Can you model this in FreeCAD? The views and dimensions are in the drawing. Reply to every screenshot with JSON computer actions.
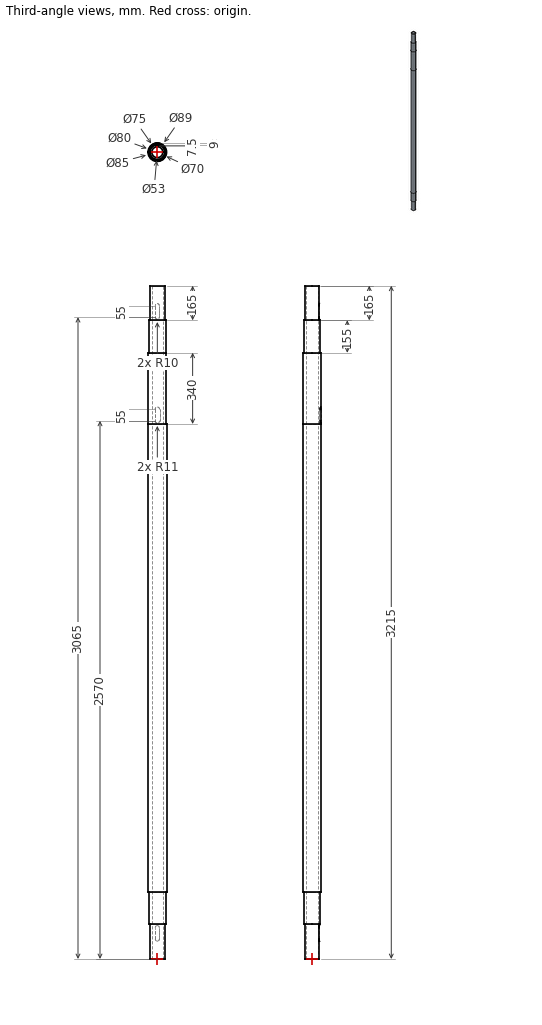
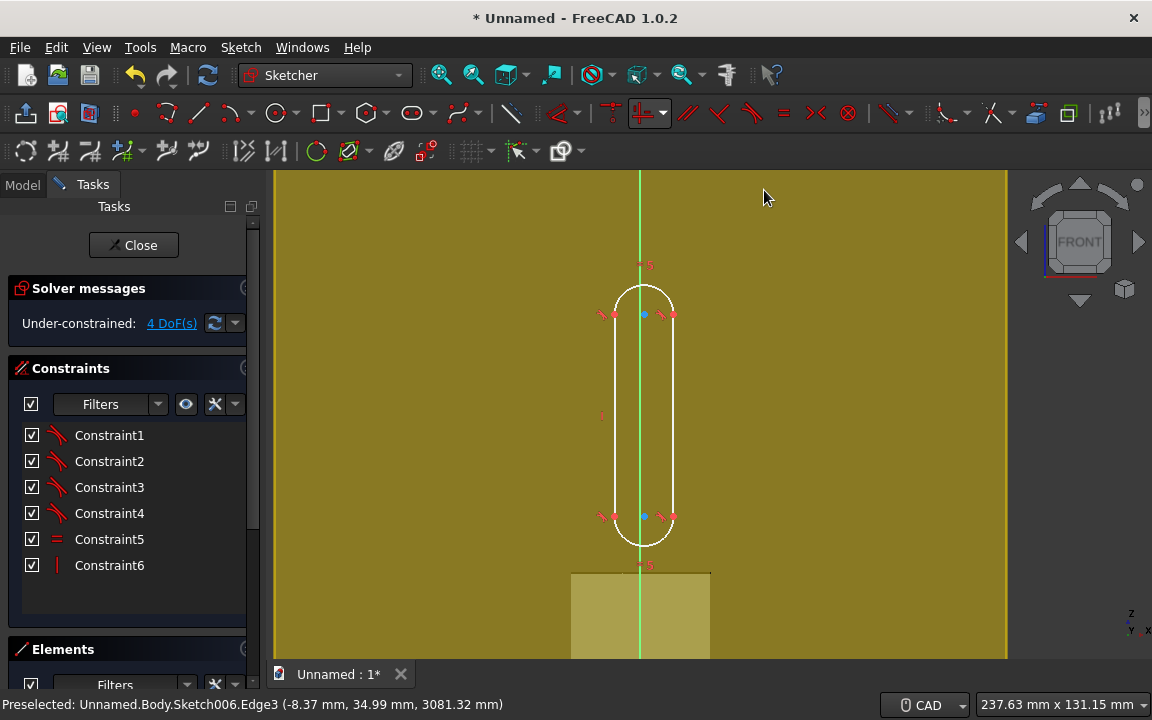
{"action": "left_click", "coordinate": [644, 517]}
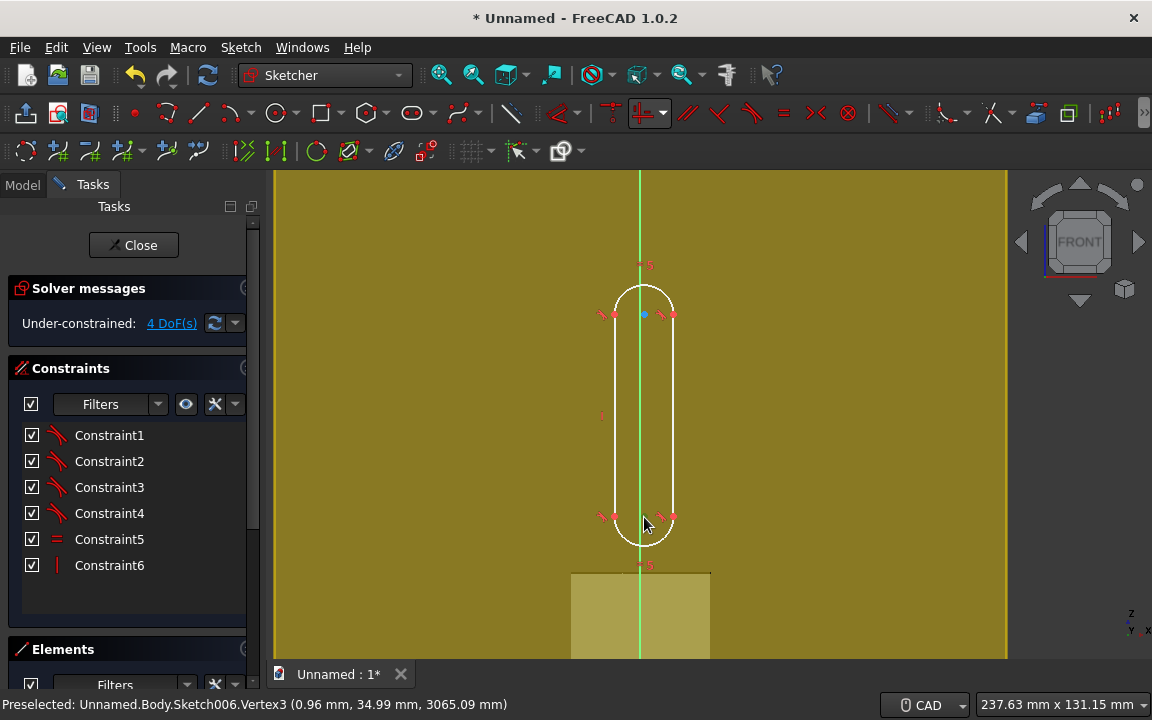
{"action": "left_click", "coordinate": [640, 600]}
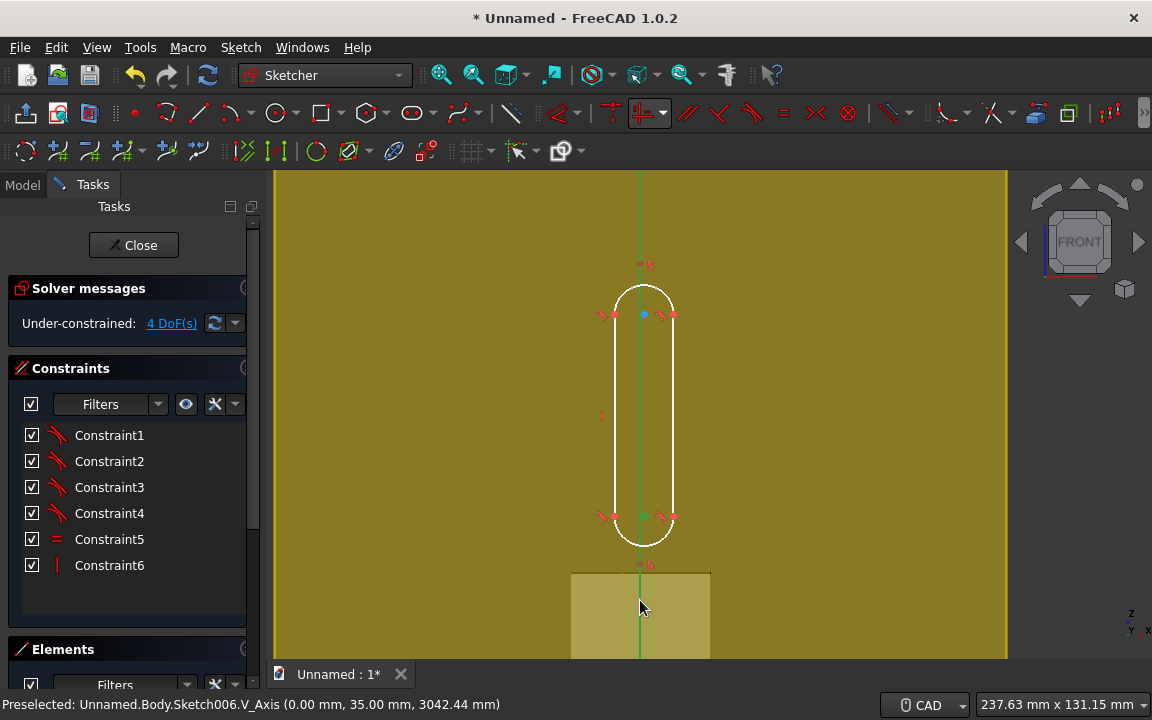
{"action": "left_click", "coordinate": [612, 114]}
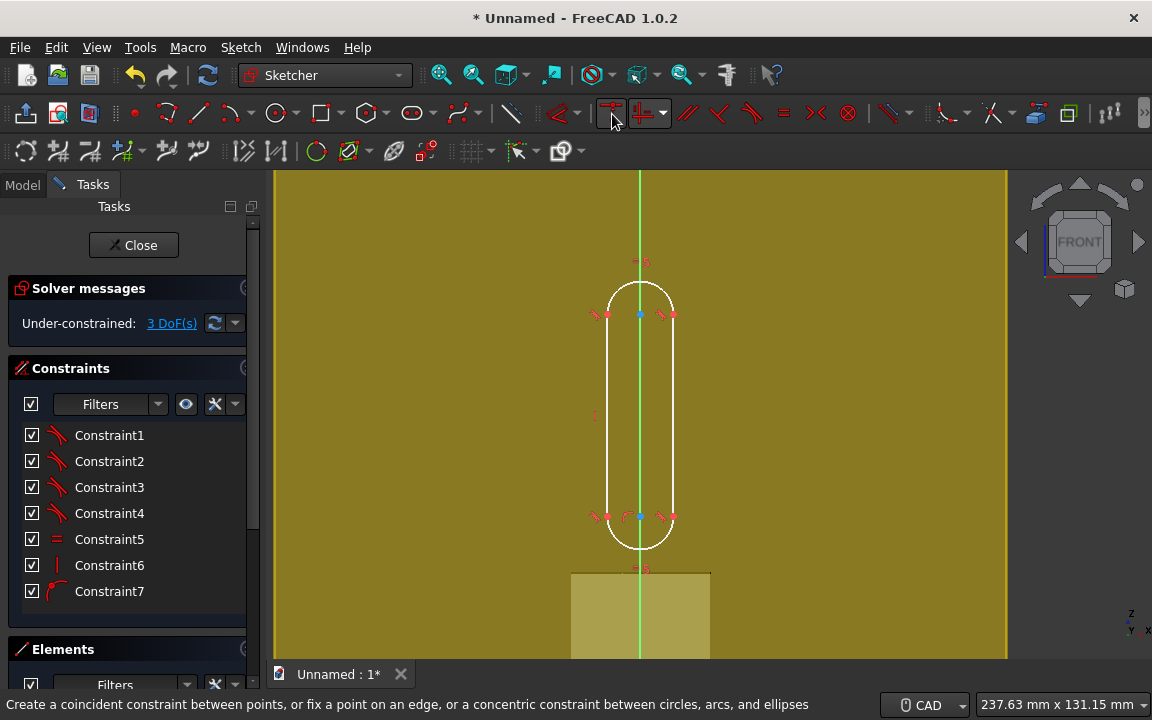
{"action": "left_click", "coordinate": [558, 114]}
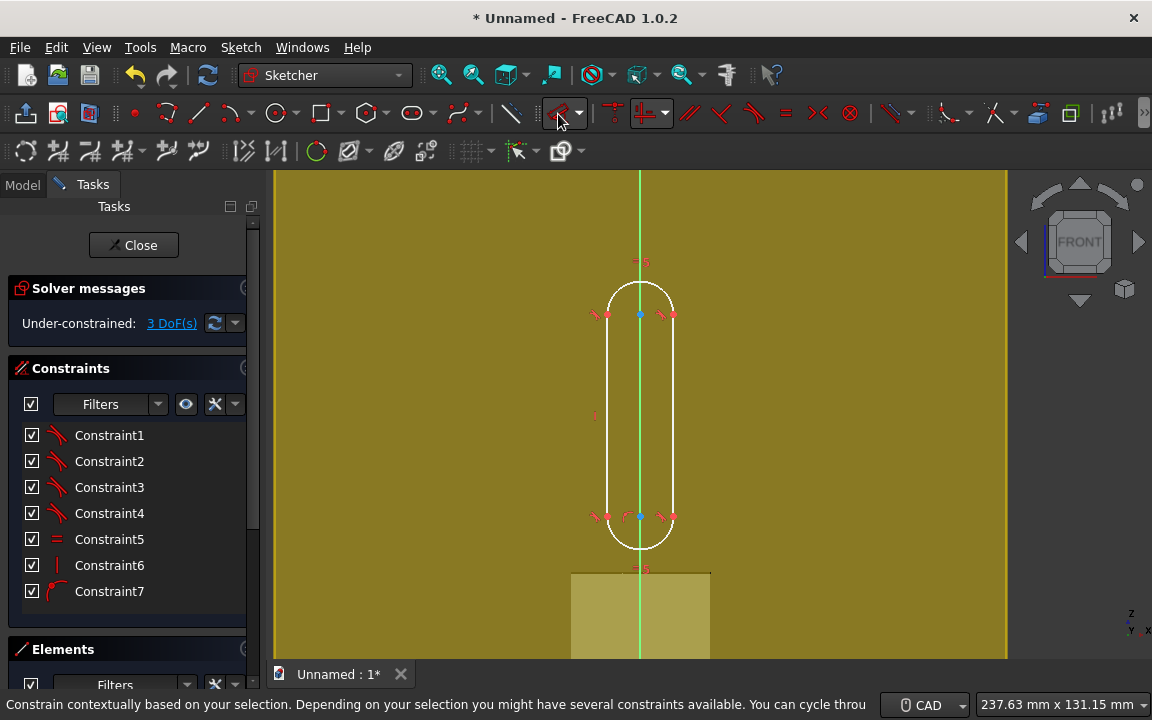
{"action": "left_click", "coordinate": [621, 543]}
{"action": "left_click", "coordinate": [602, 569]}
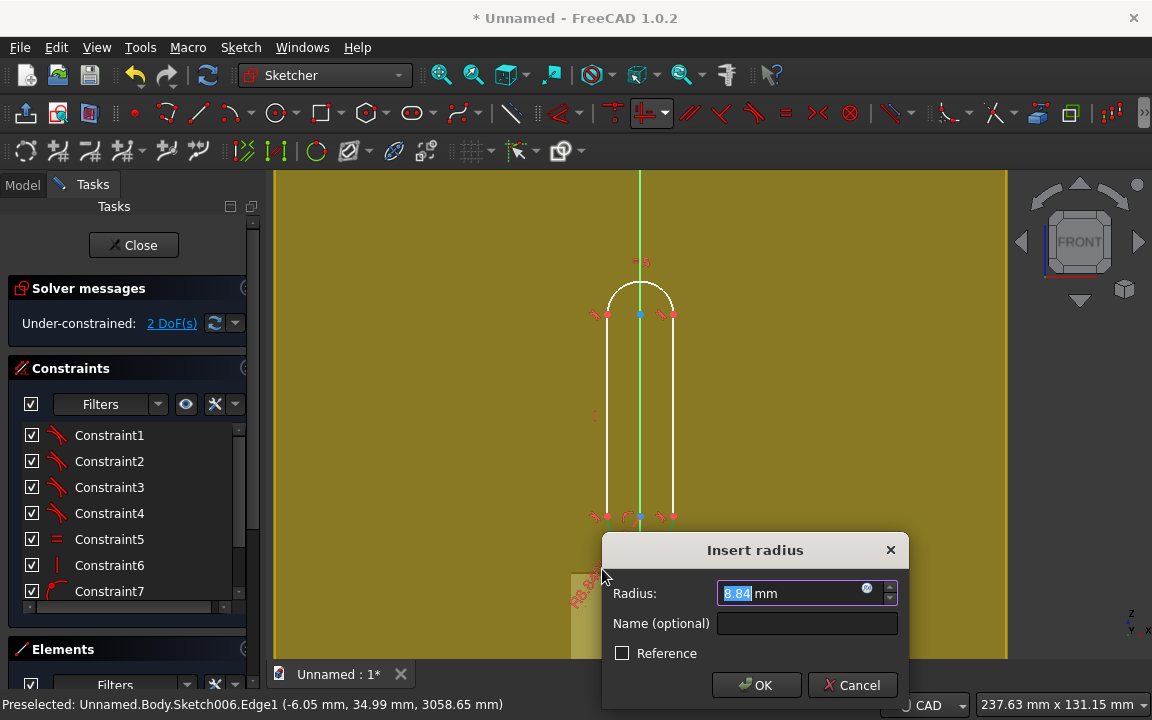
{"action": "type", "text": "10"}
{"action": "key", "text": "Return"}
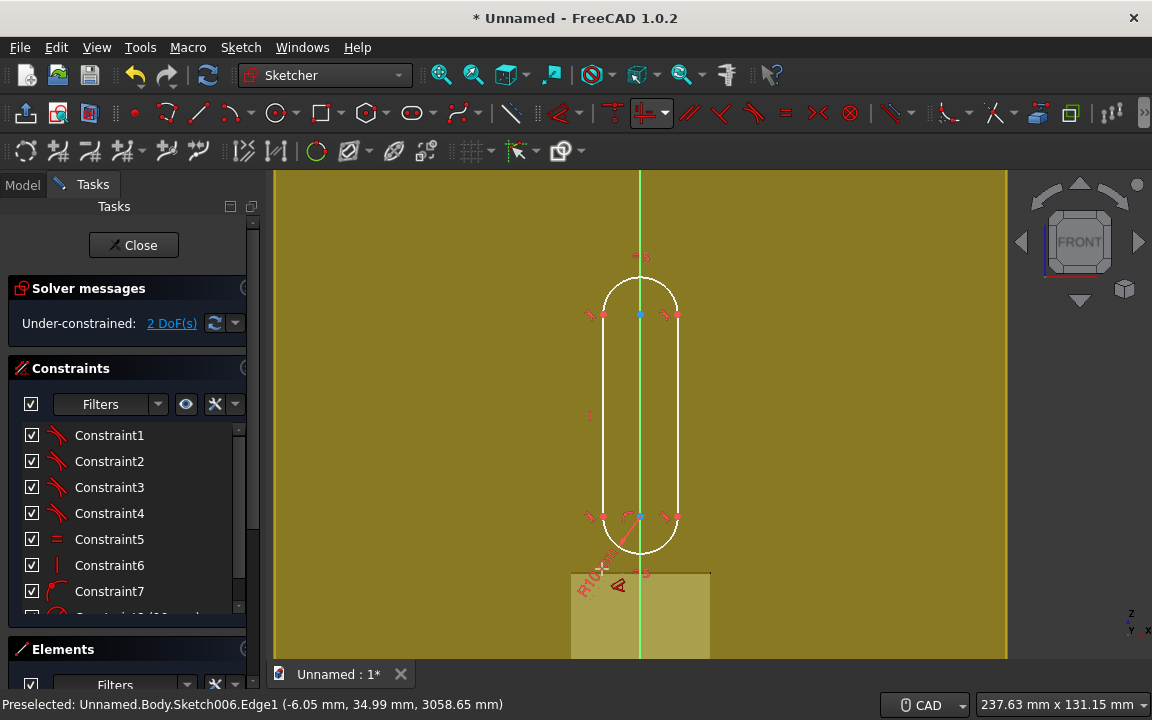
{"action": "left_click", "coordinate": [603, 456]}
{"action": "left_click", "coordinate": [569, 416]}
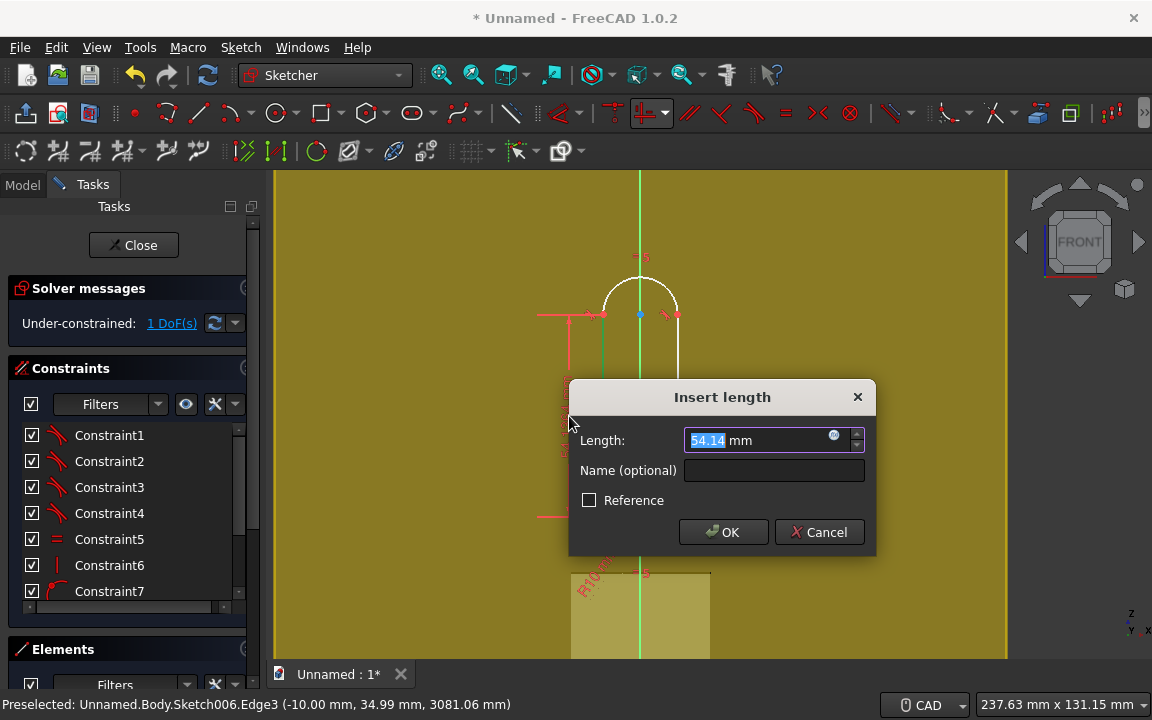
{"action": "type", "text": "55"}
{"action": "key", "text": "Return"}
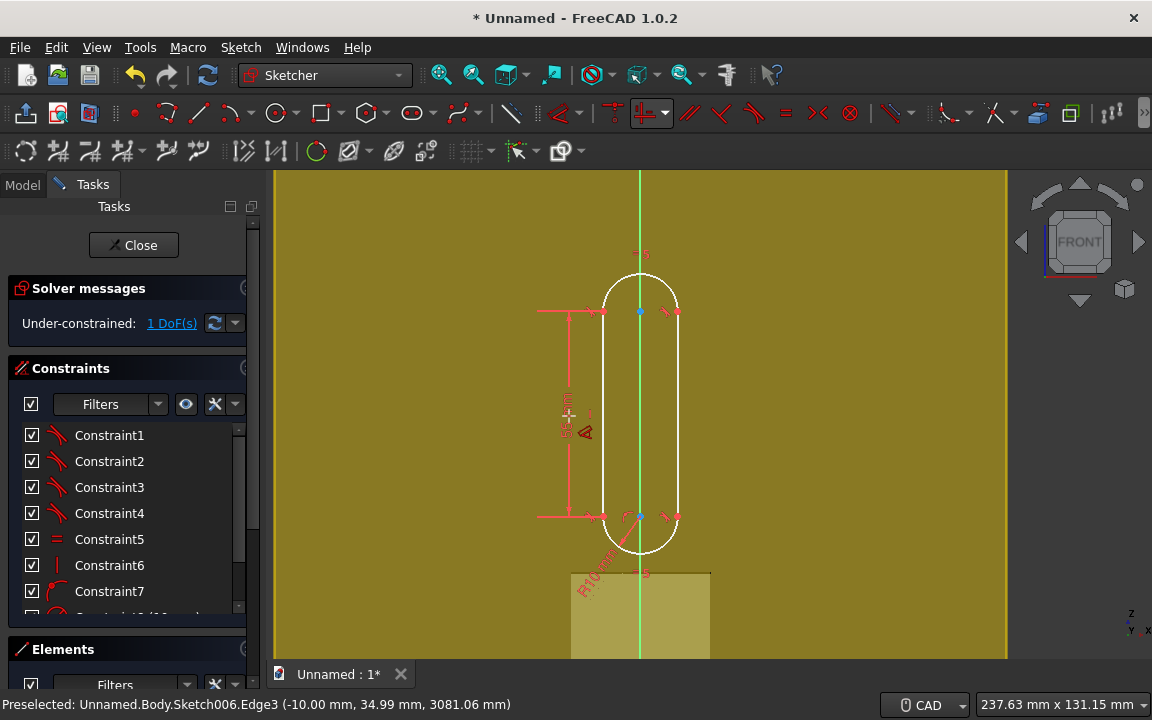
{"action": "left_click", "coordinate": [603, 517]}
{"action": "left_click", "coordinate": [569, 547]}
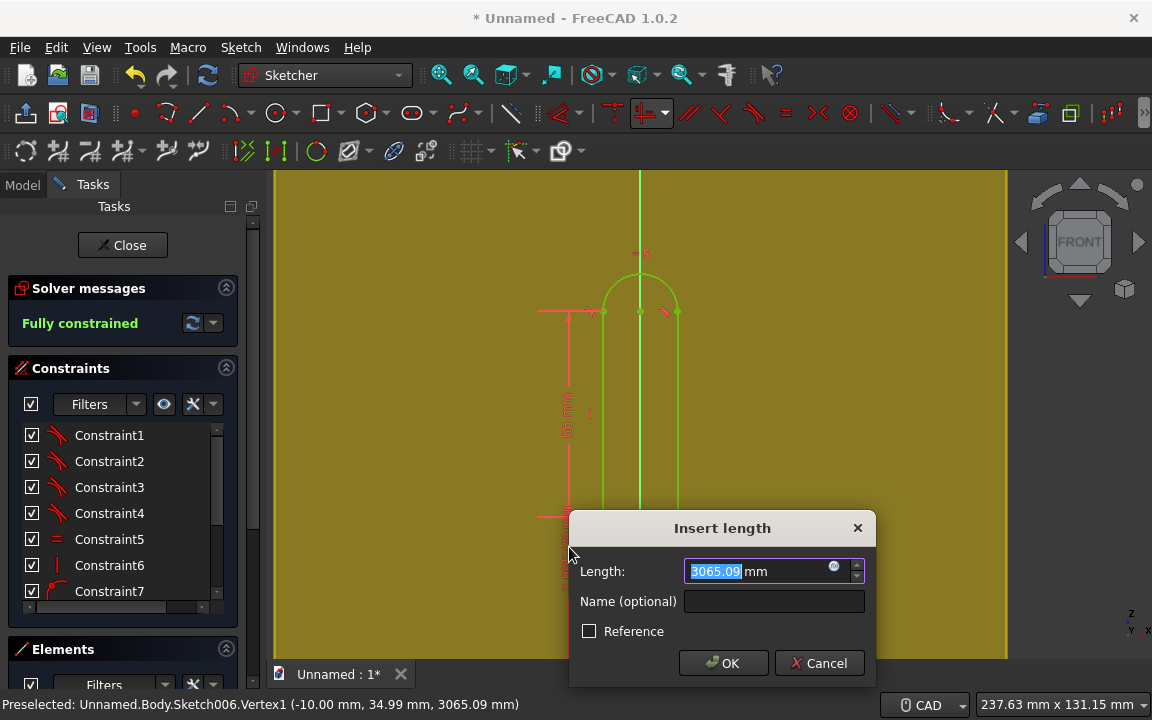
{"action": "type", "text": "3065"}
{"action": "key", "text": "Return"}
{"action": "key", "text": "Escape"}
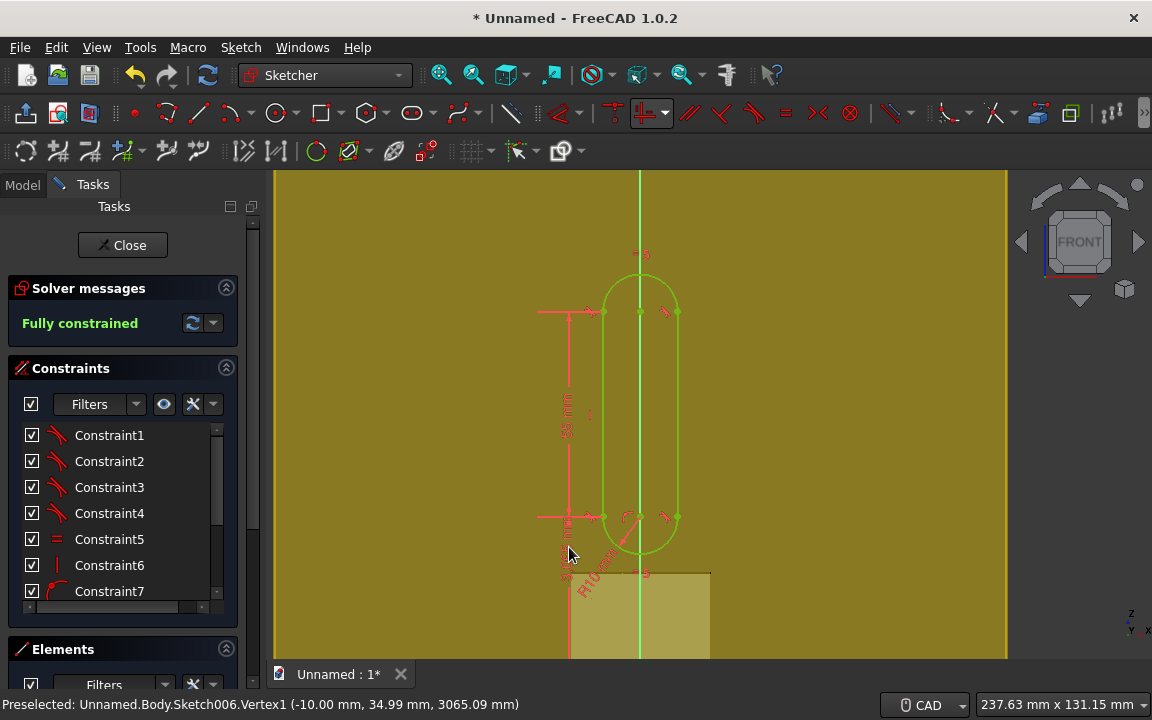
{"action": "left_click", "coordinate": [123, 245]}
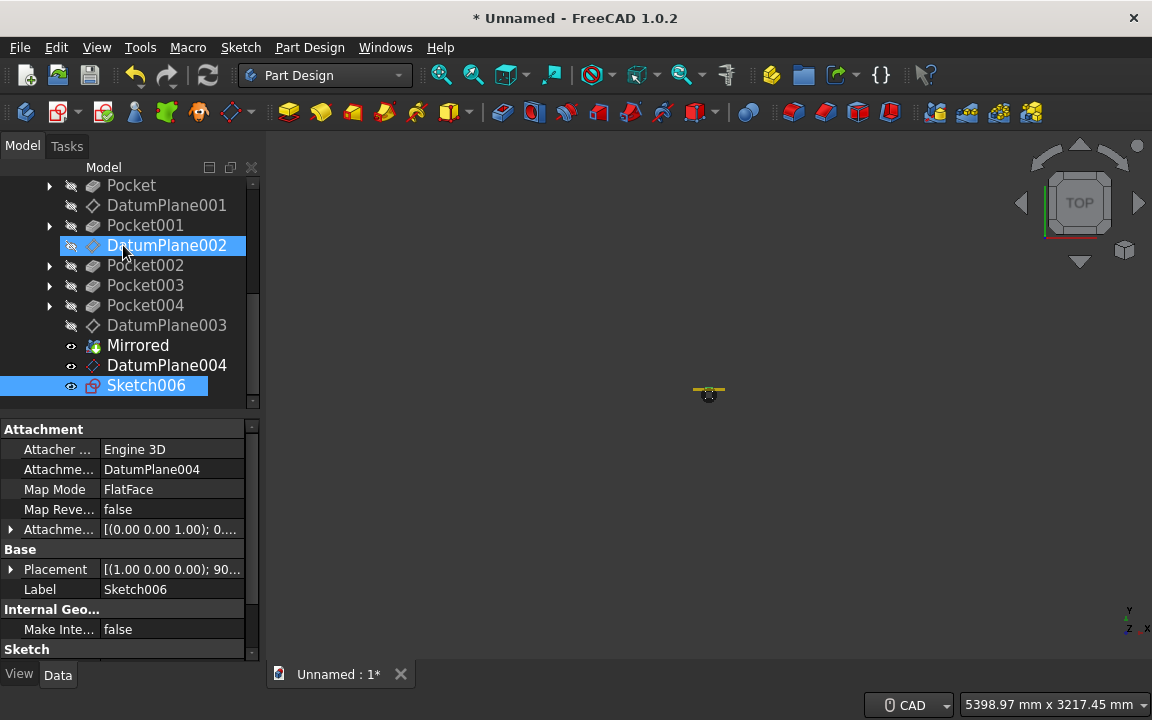
{"action": "left_click", "coordinate": [504, 112]}